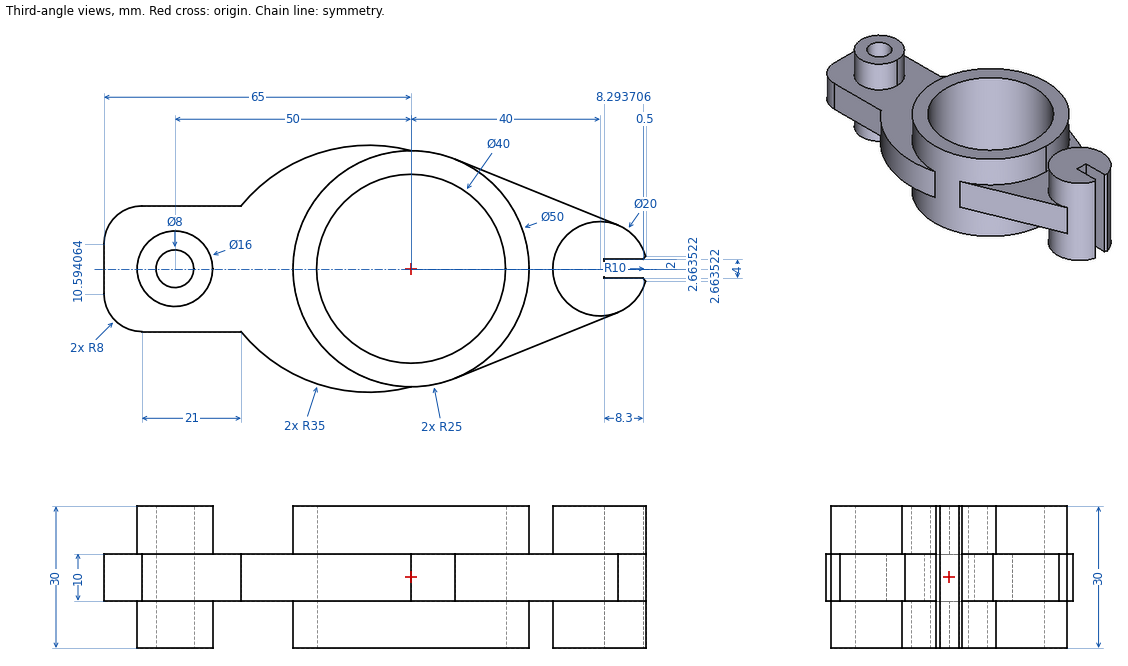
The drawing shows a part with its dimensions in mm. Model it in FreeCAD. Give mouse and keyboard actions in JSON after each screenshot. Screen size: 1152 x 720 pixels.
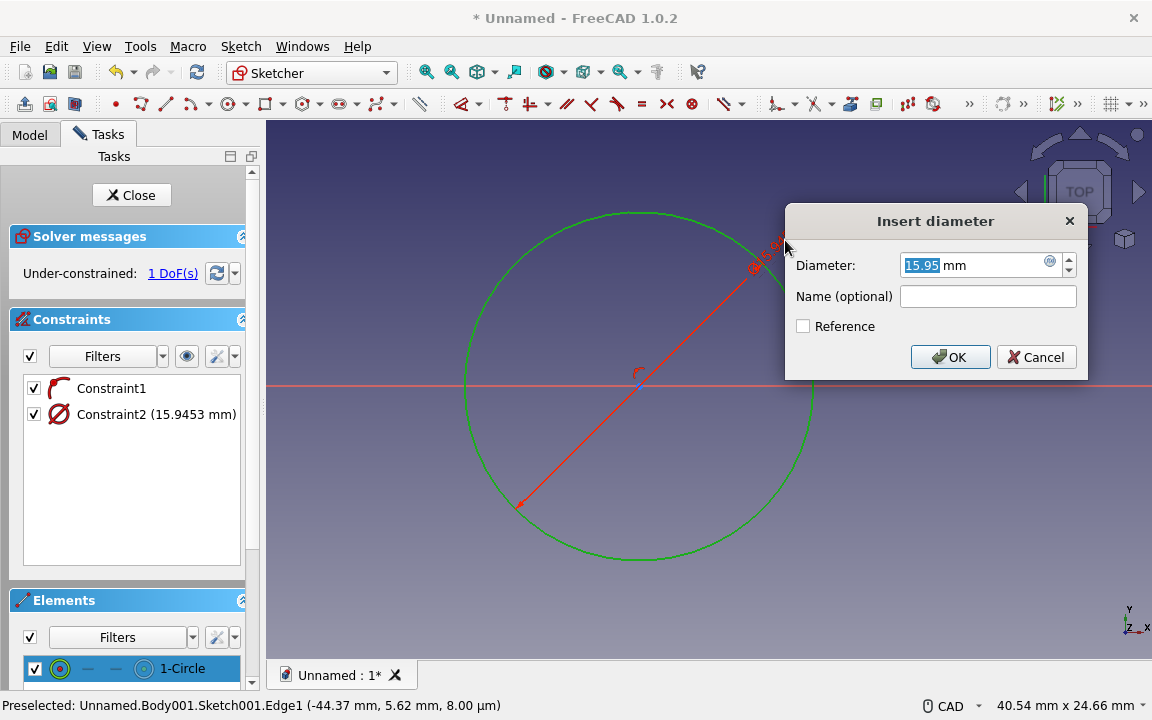
{"action": "type", "text": "16"}
{"action": "key", "text": "Return"}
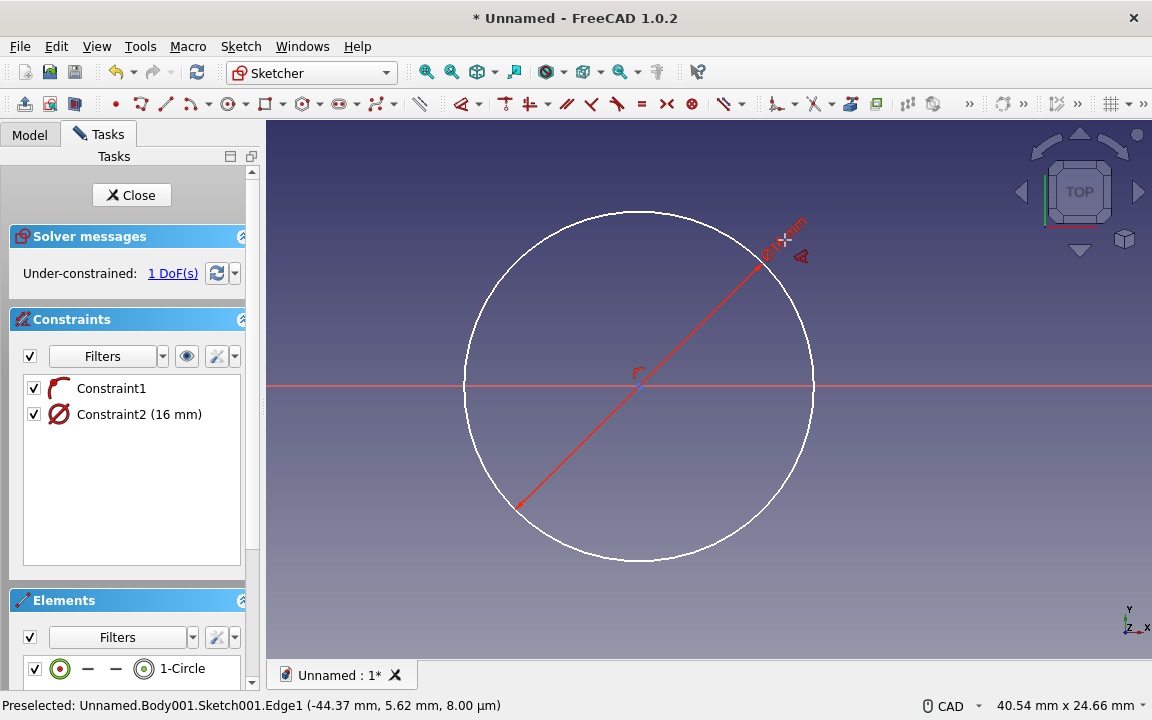
{"action": "left_click", "coordinate": [639, 386]}
{"action": "left_click", "coordinate": [733, 420]}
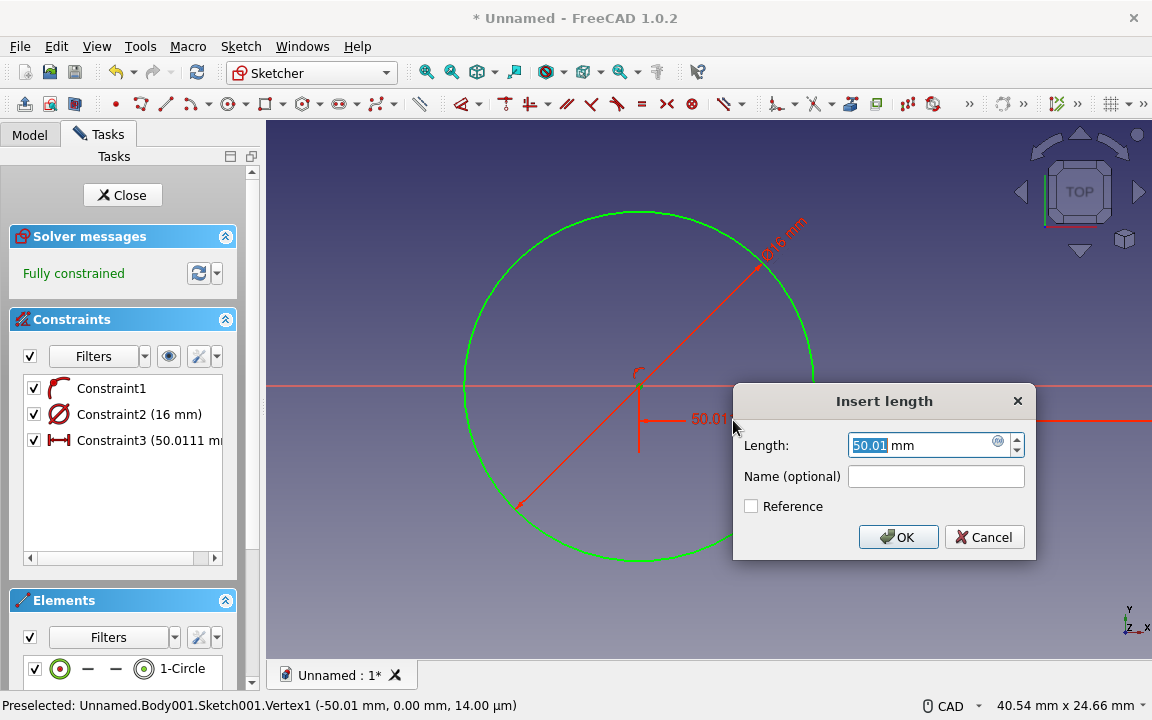
{"action": "type", "text": "50"}
{"action": "key", "text": "Return"}
{"action": "key", "text": "Escape"}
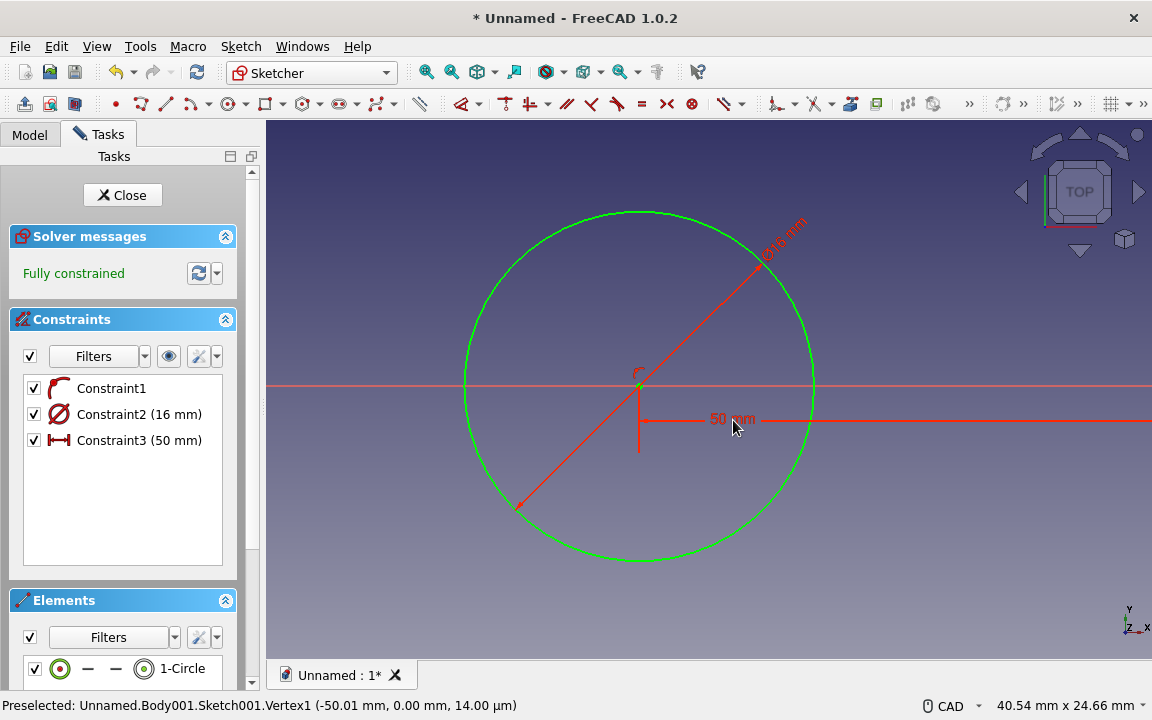
{"action": "left_click", "coordinate": [123, 195]}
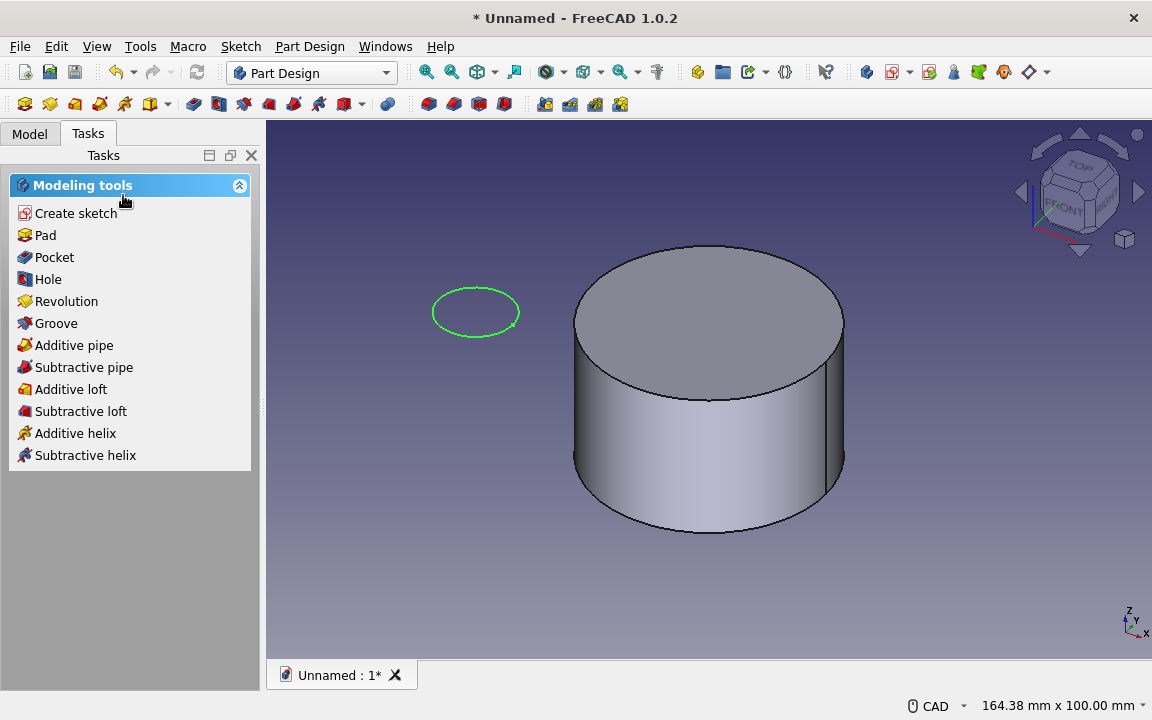
{"action": "left_click", "coordinate": [25, 104]}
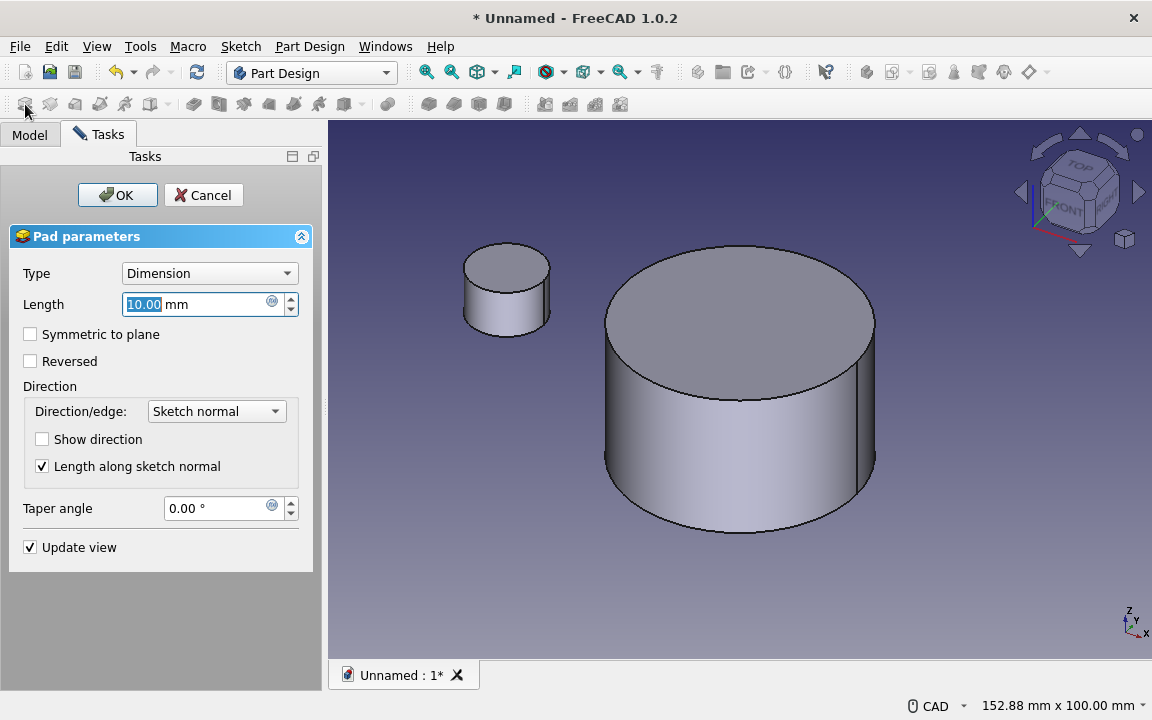
{"action": "type", "text": "30"}
{"action": "key", "text": "Tab"}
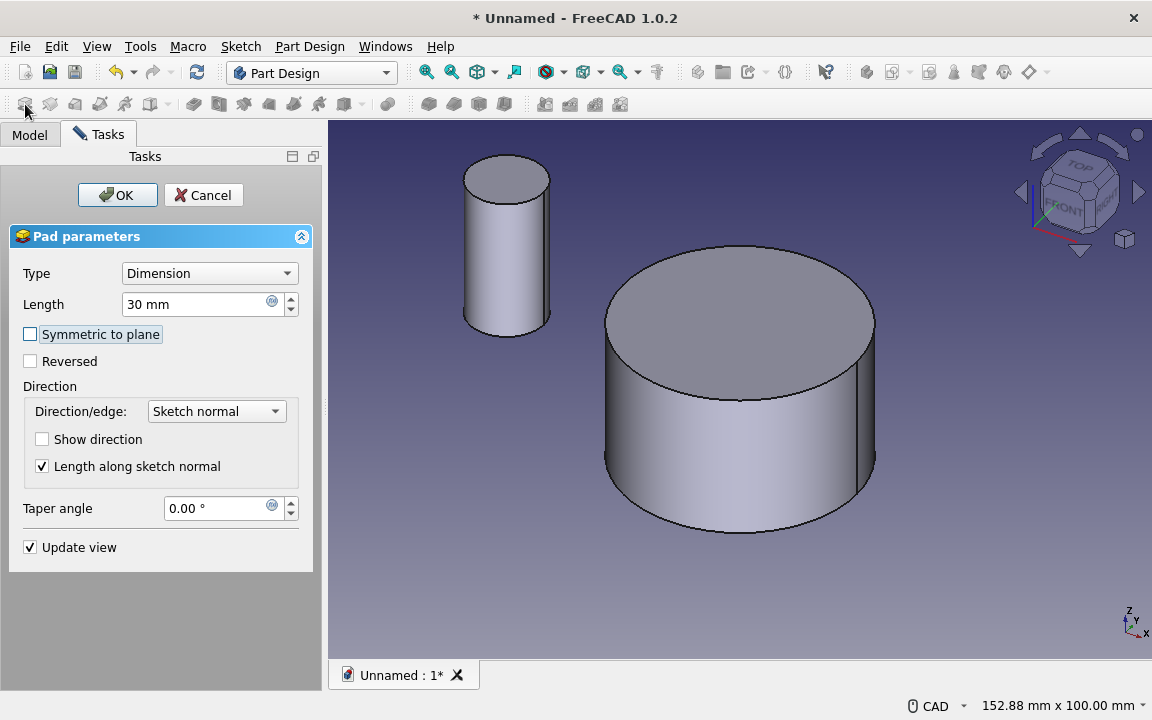
{"action": "left_click", "coordinate": [31, 334]}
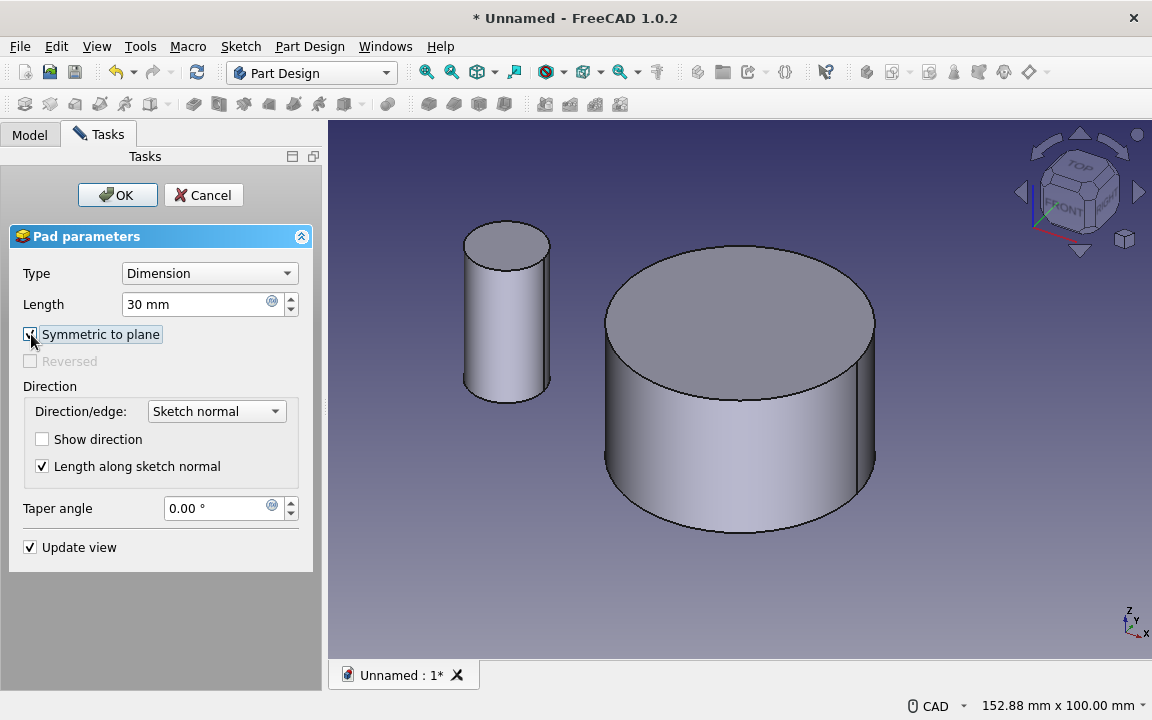
{"action": "left_click", "coordinate": [118, 195]}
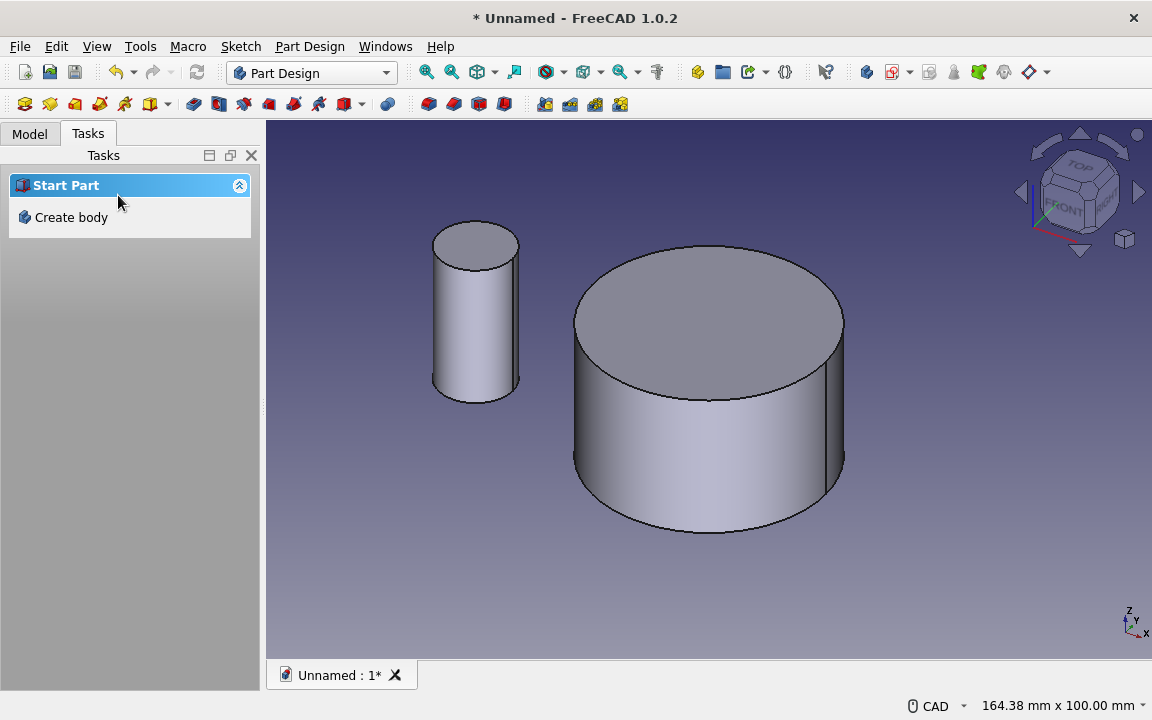
{"action": "left_click", "coordinate": [427, 72]}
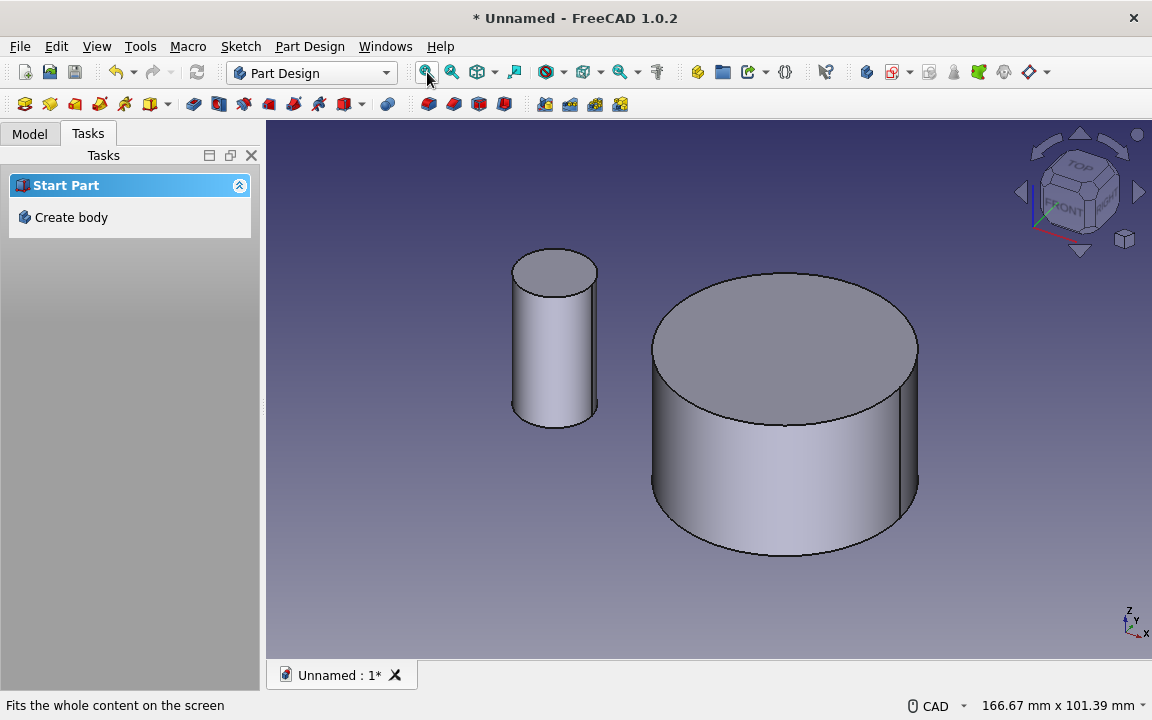
{"action": "left_click", "coordinate": [867, 72]}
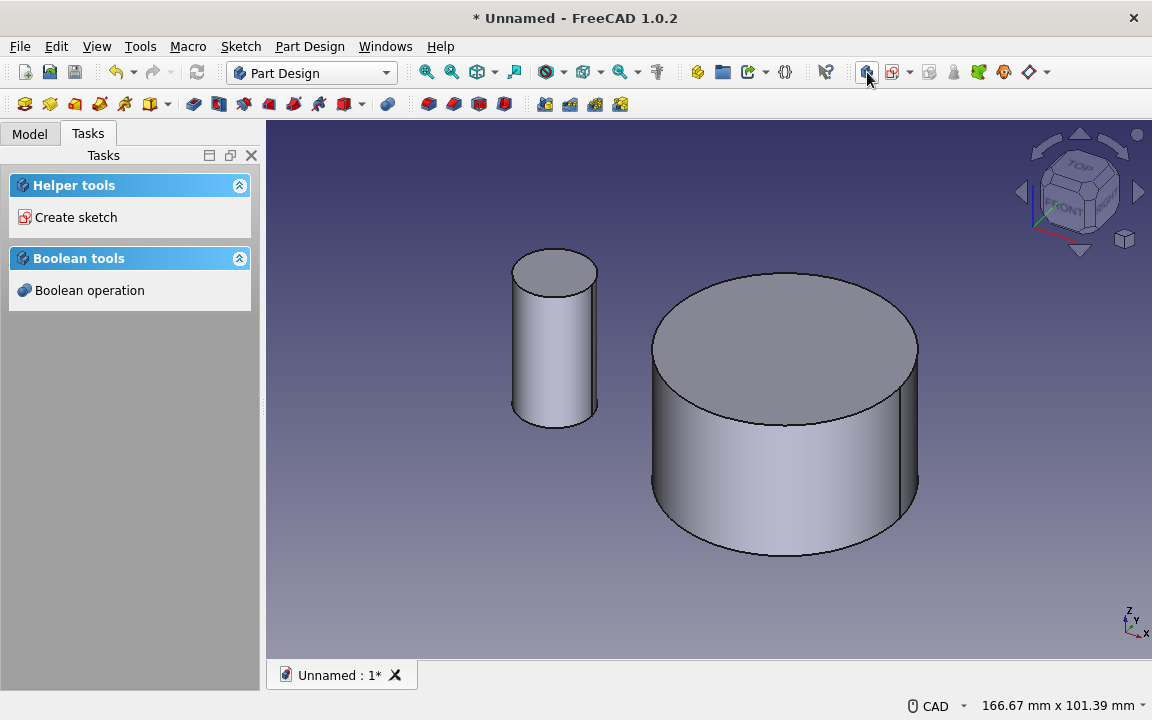
{"action": "left_click", "coordinate": [306, 619]}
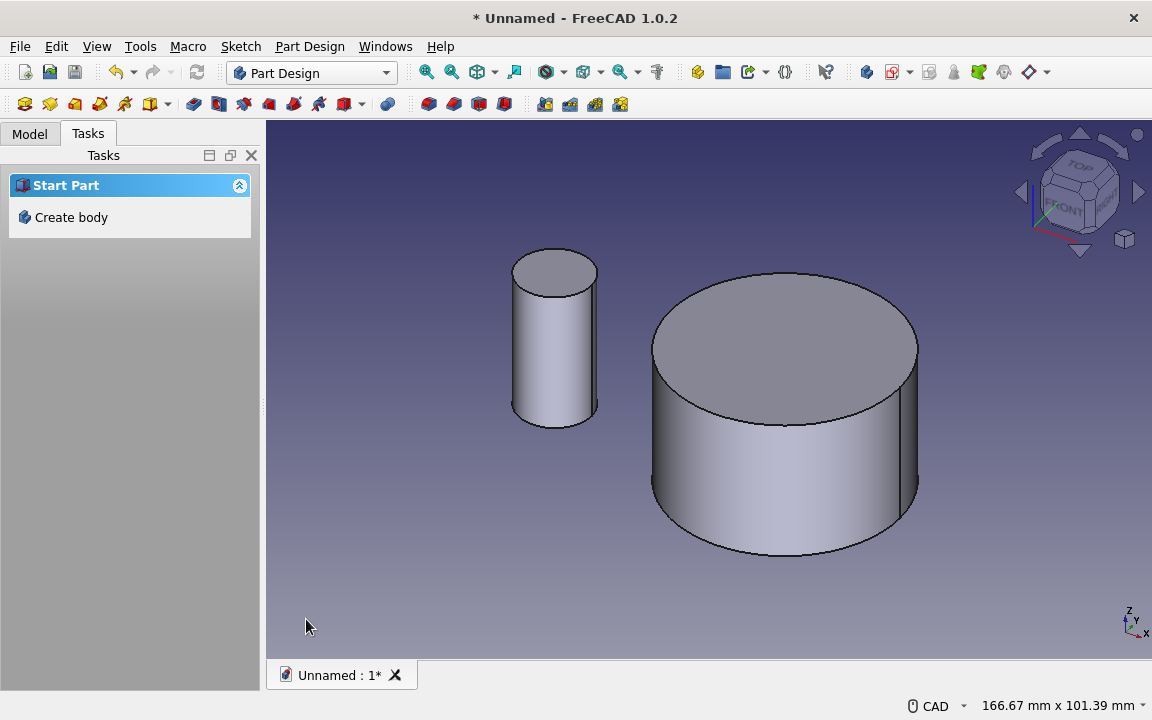
{"action": "left_click", "coordinate": [892, 72]}